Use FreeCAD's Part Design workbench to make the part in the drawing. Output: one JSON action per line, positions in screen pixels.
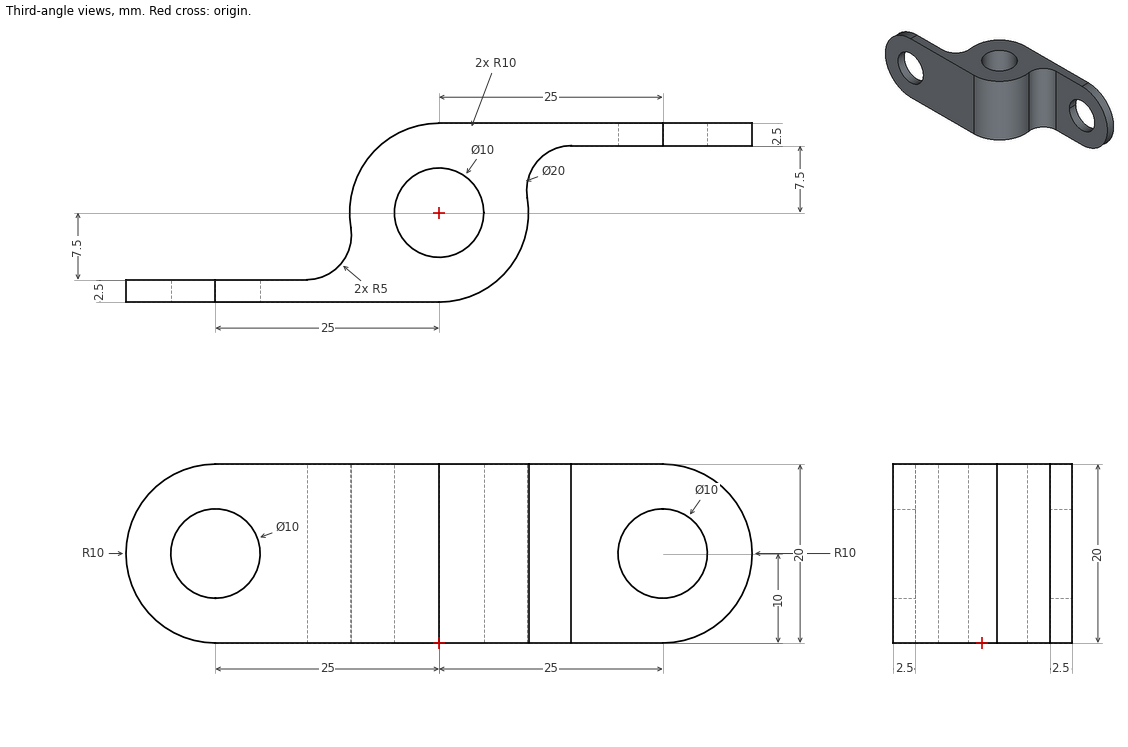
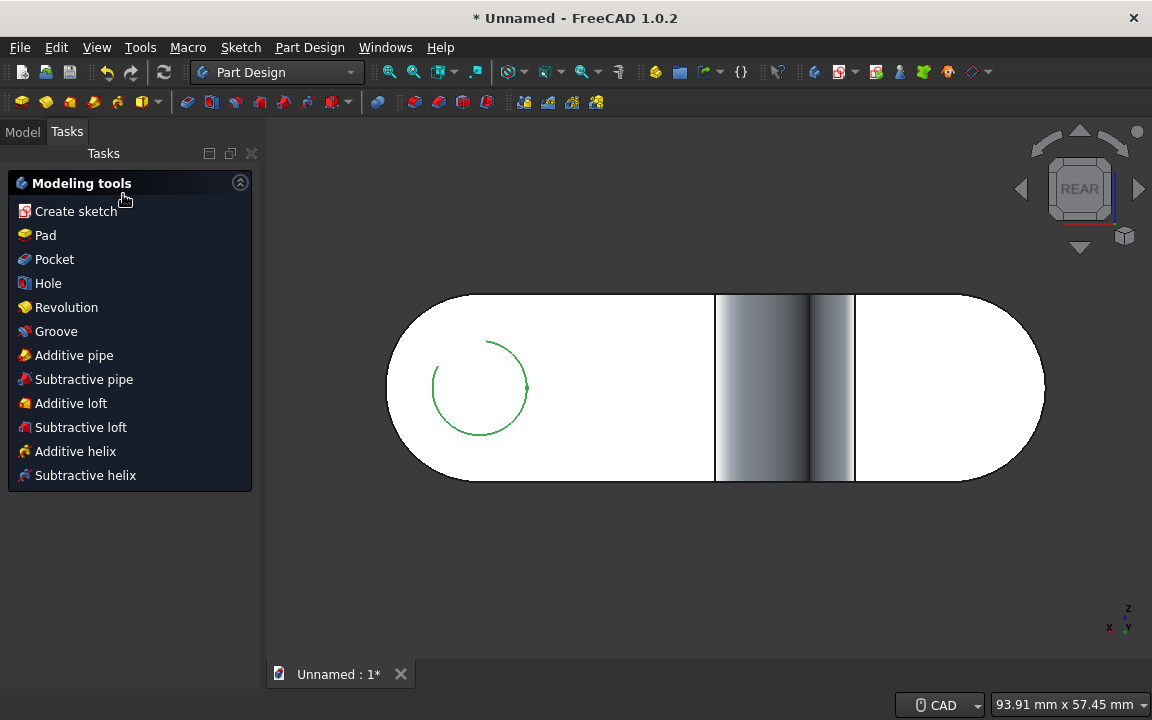
{"action": "left_click", "coordinate": [188, 102]}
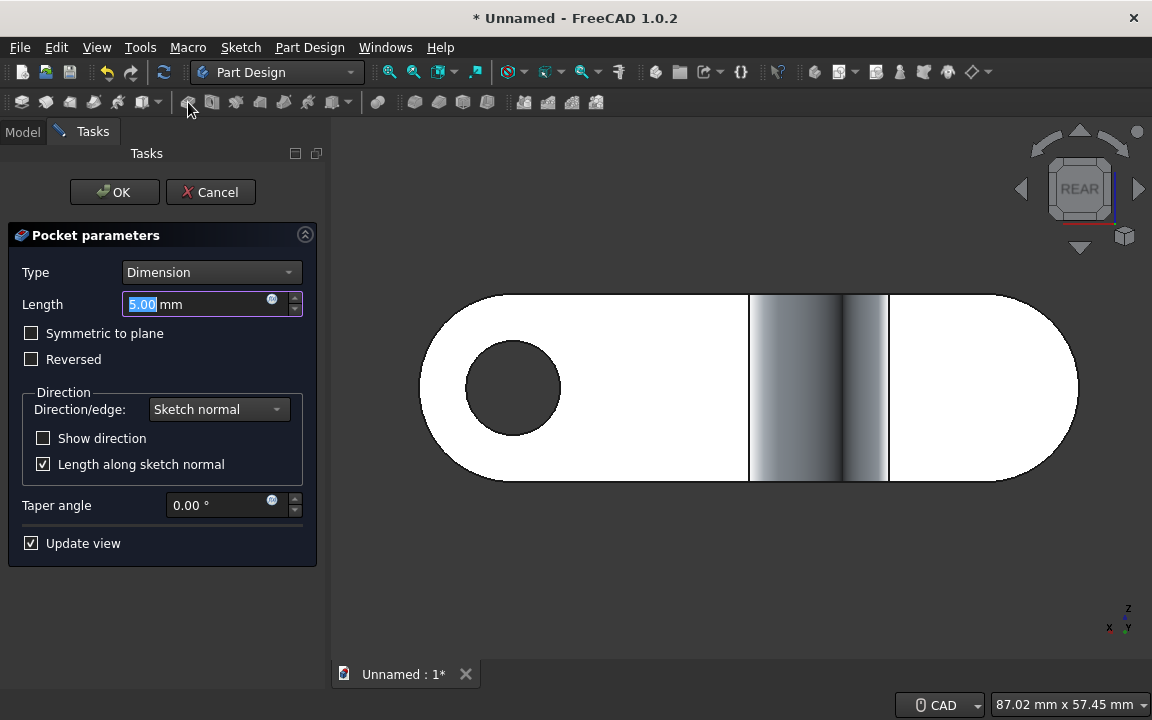
{"action": "type", "text": "2.5"}
{"action": "key", "text": "Tab"}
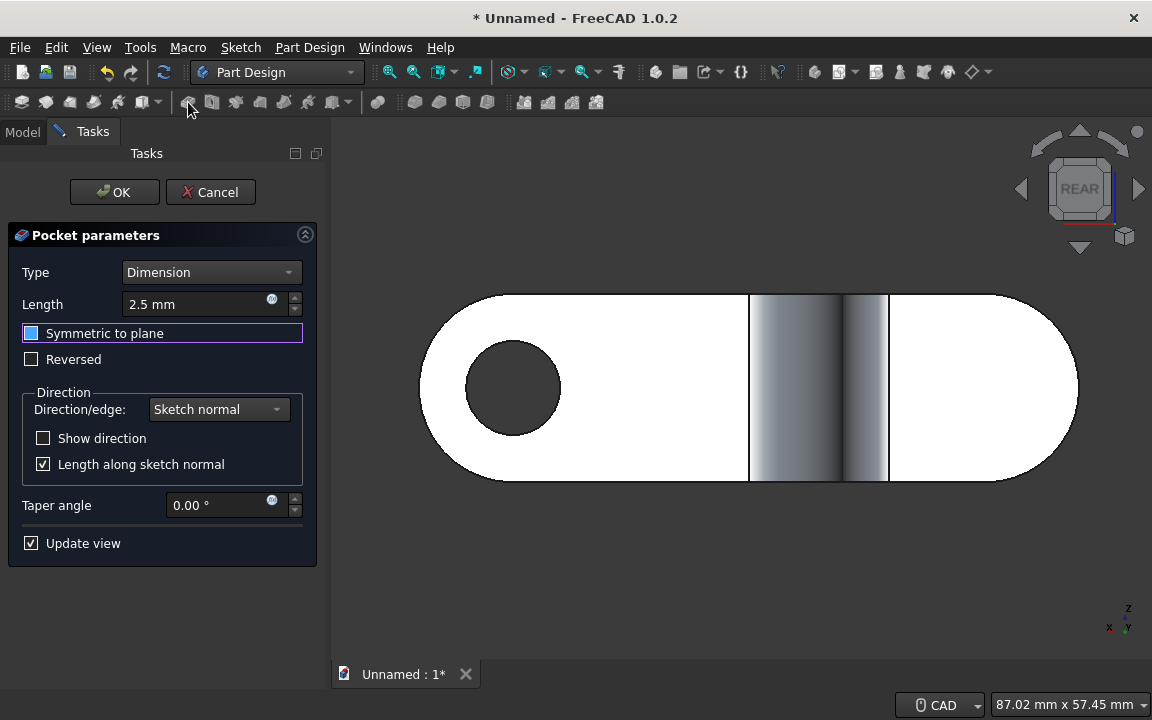
{"action": "left_click", "coordinate": [115, 192]}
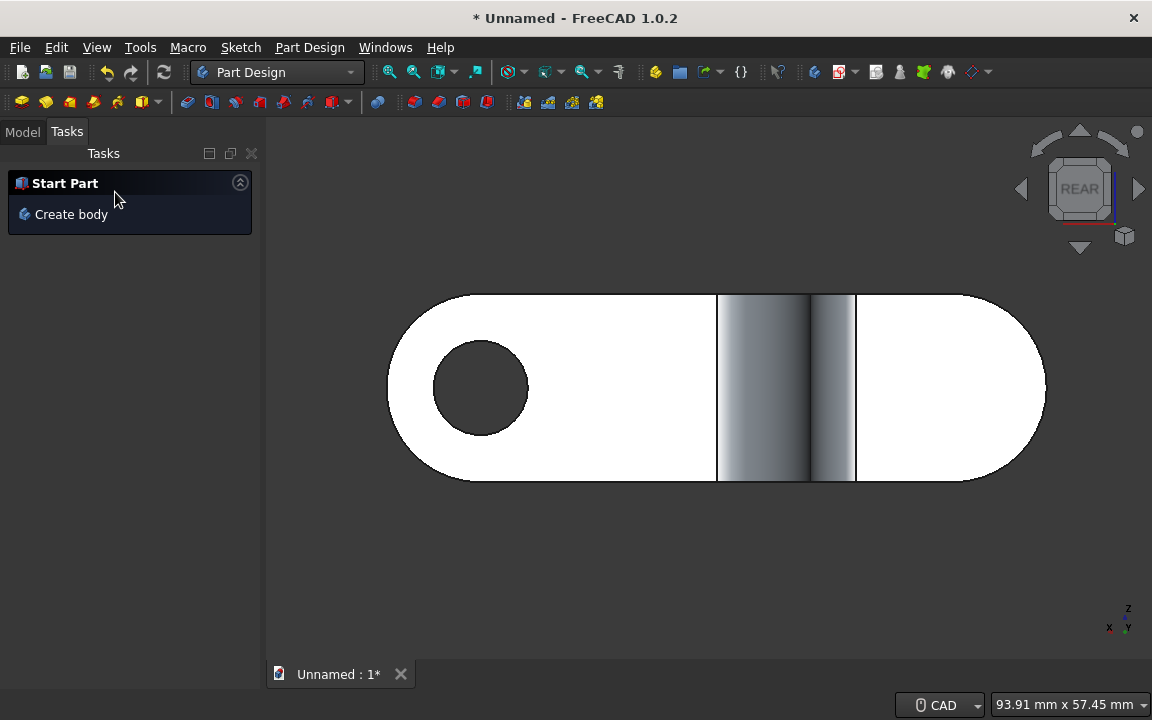
{"action": "key", "text": "0"}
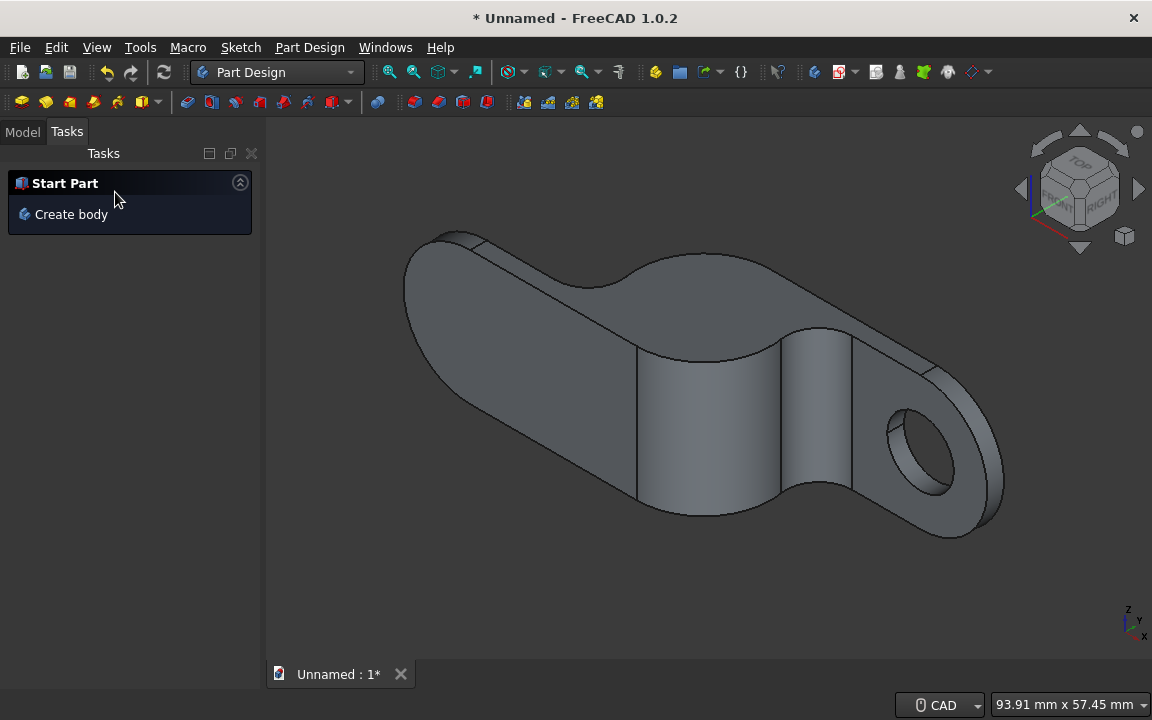
{"action": "left_click", "coordinate": [554, 374]}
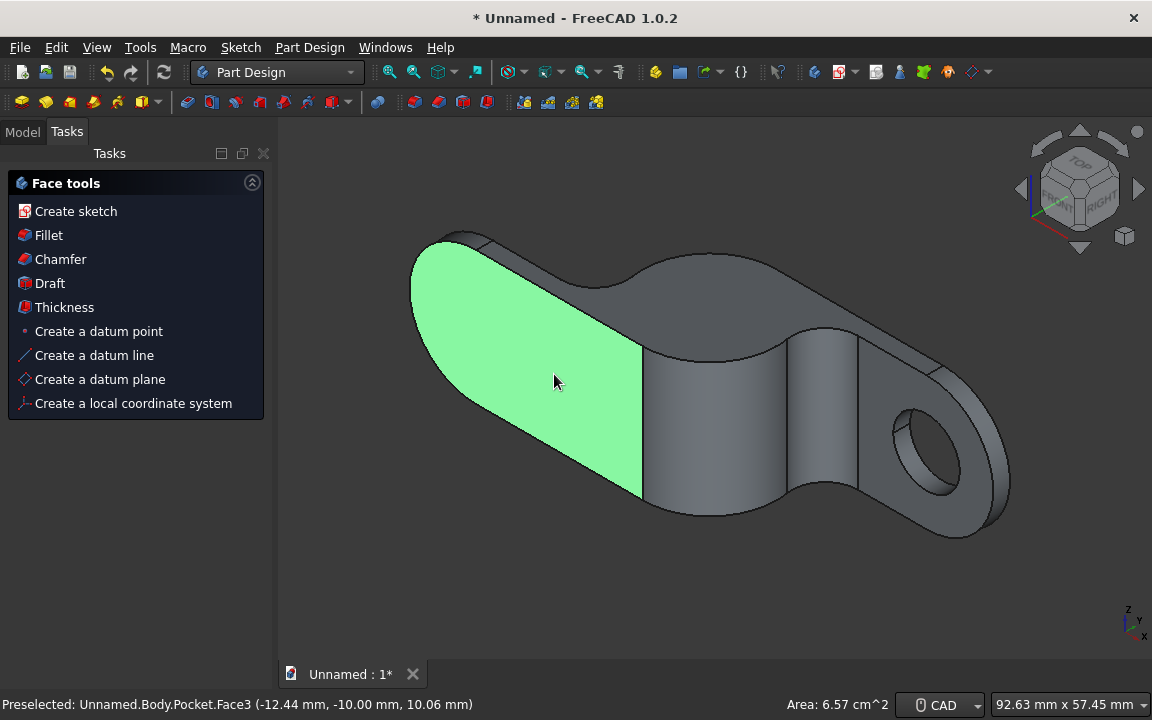
{"action": "left_click", "coordinate": [840, 72]}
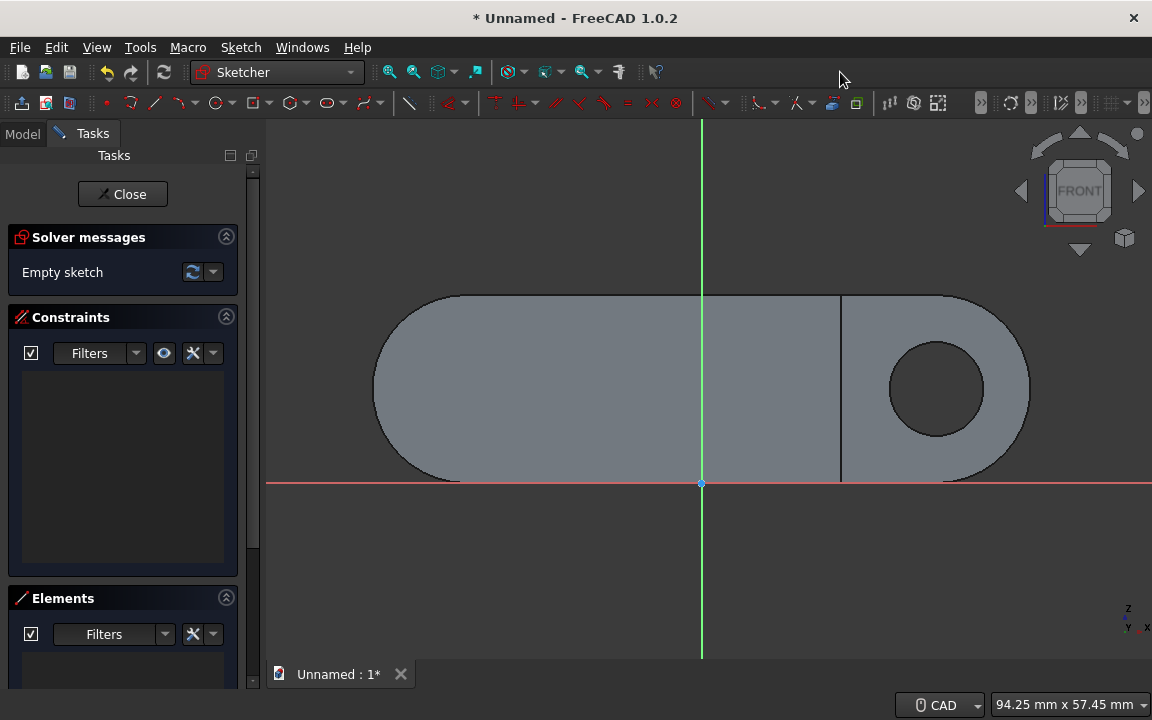
{"action": "scroll", "coordinate": [392, 389], "scroll_direction": "up", "scroll_amount": 6}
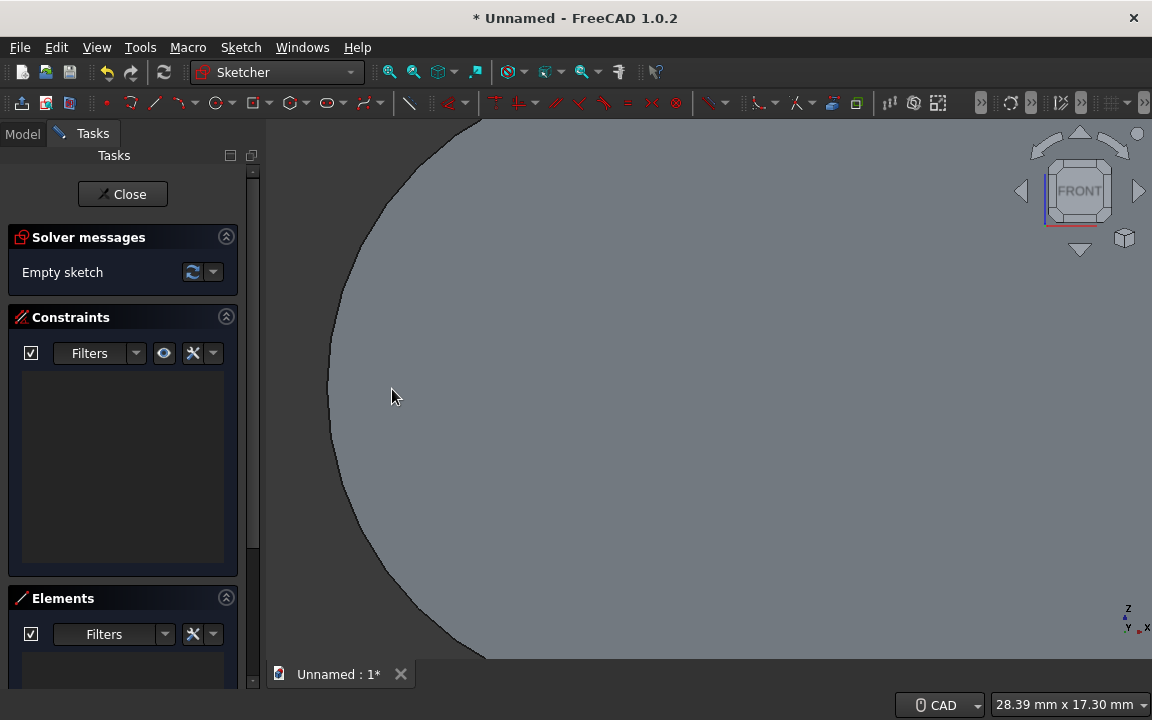
{"action": "left_click", "coordinate": [216, 104]}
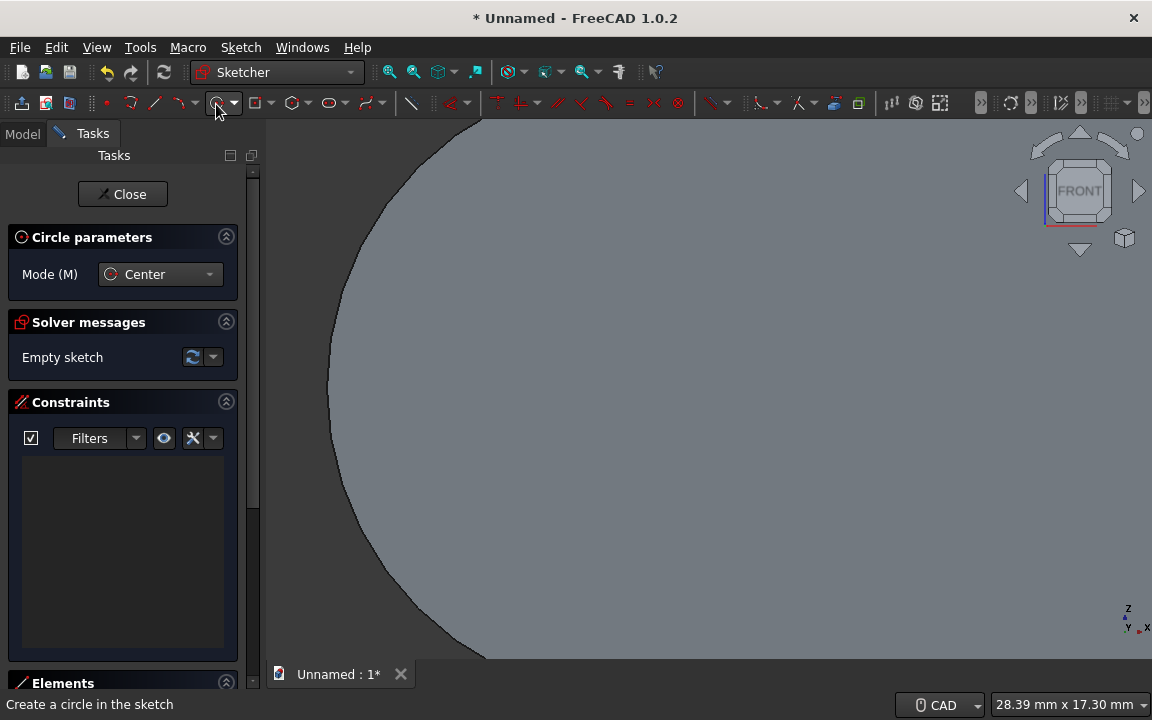
{"action": "left_click", "coordinate": [639, 388]}
{"action": "left_click", "coordinate": [749, 277]}
{"action": "key", "text": "Escape"}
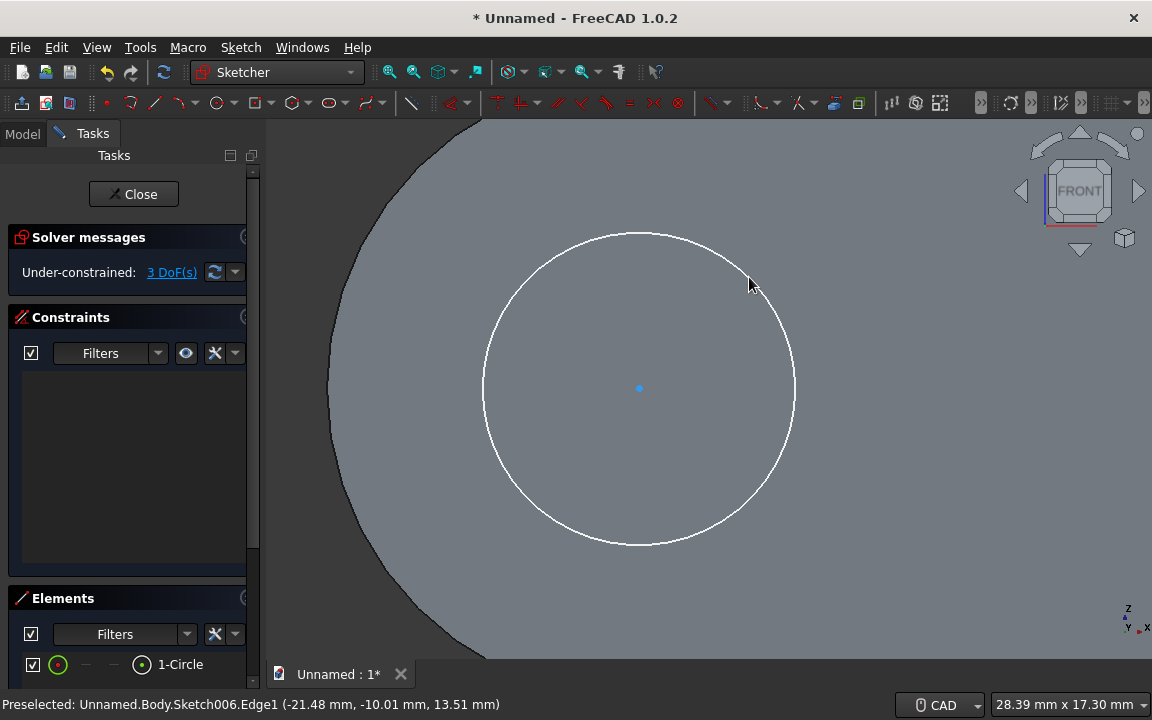
{"action": "key", "text": "d"}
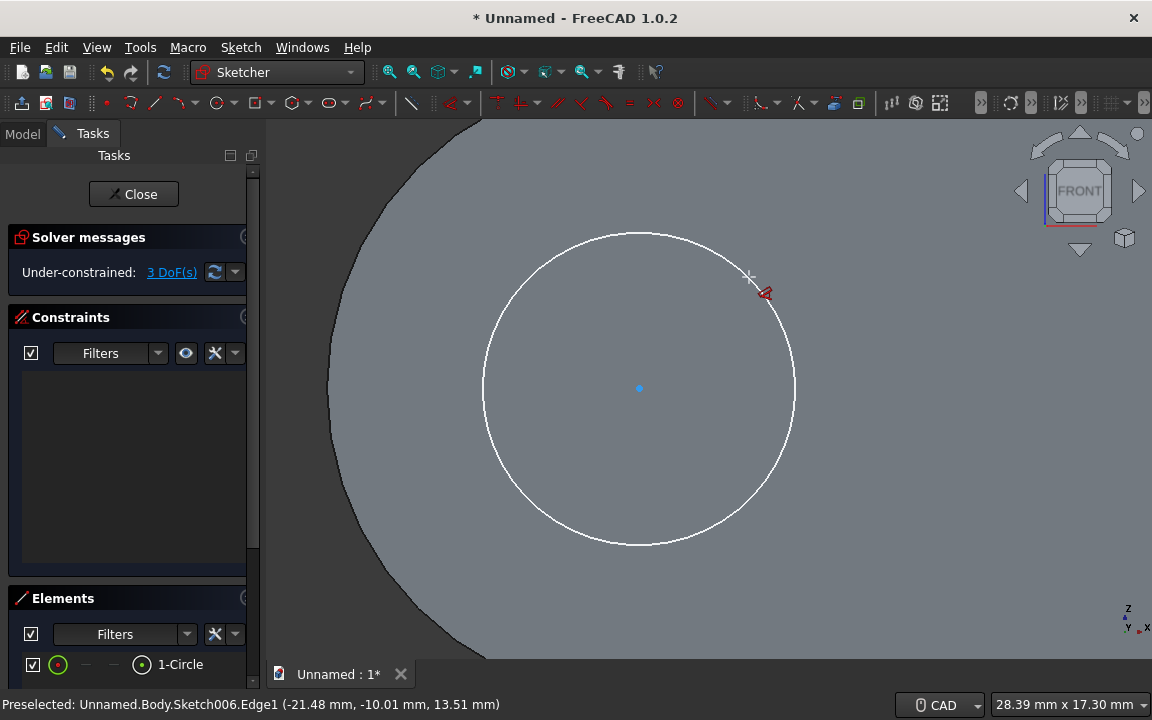
{"action": "left_click", "coordinate": [749, 278]}
{"action": "left_click", "coordinate": [772, 255]}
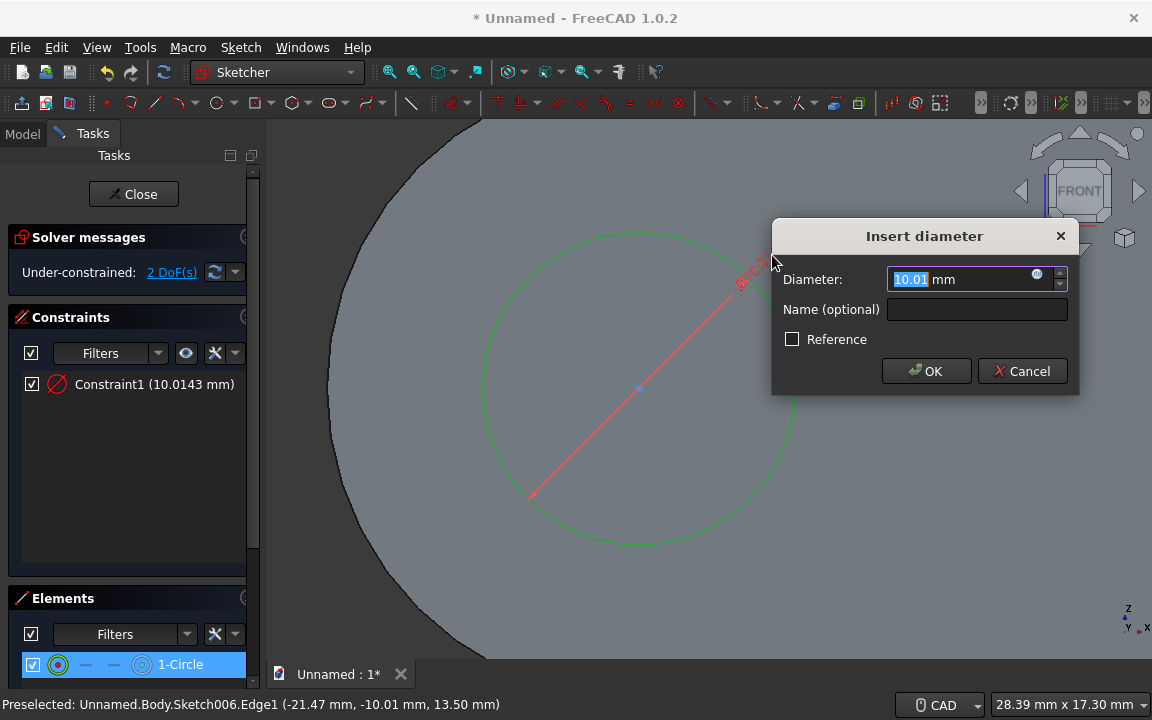
{"action": "type", "text": "10"}
{"action": "key", "text": "Return"}